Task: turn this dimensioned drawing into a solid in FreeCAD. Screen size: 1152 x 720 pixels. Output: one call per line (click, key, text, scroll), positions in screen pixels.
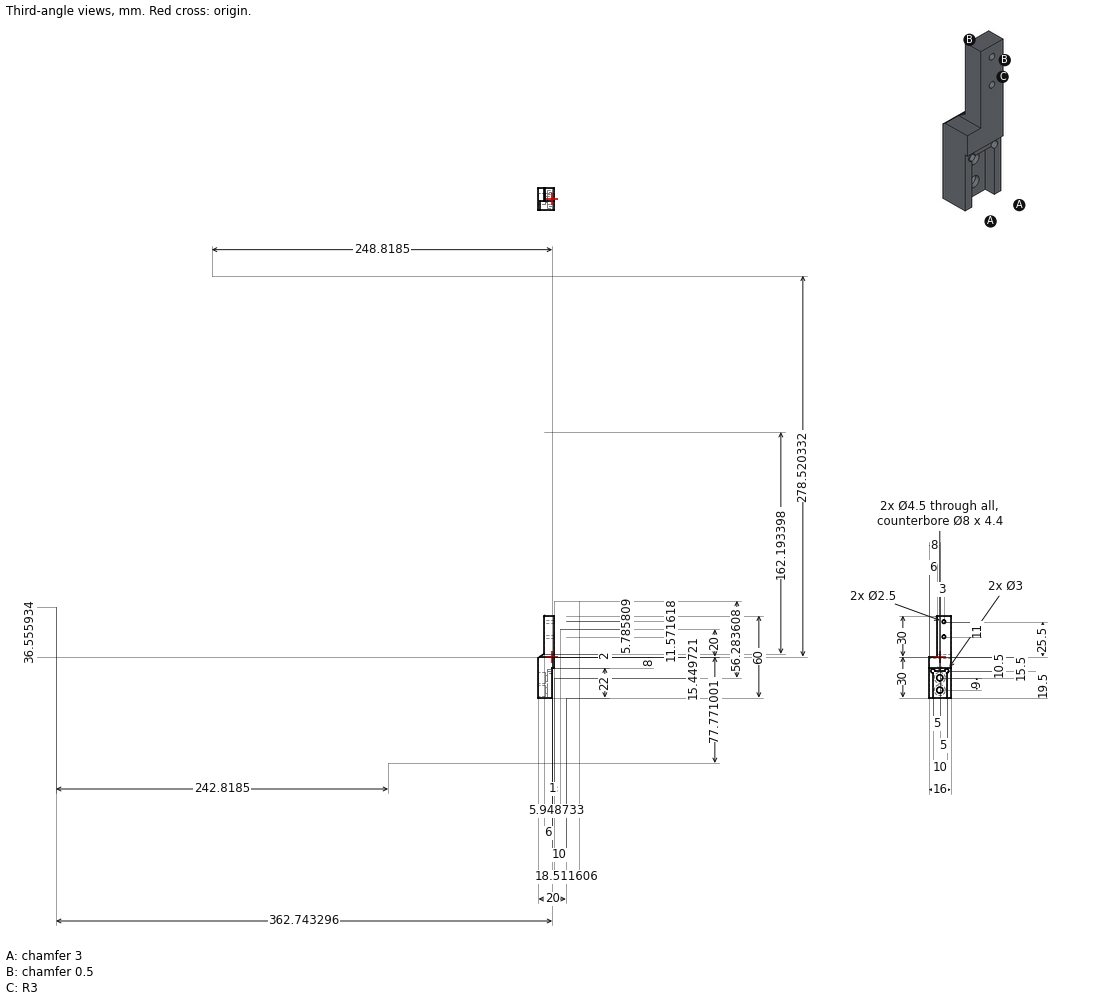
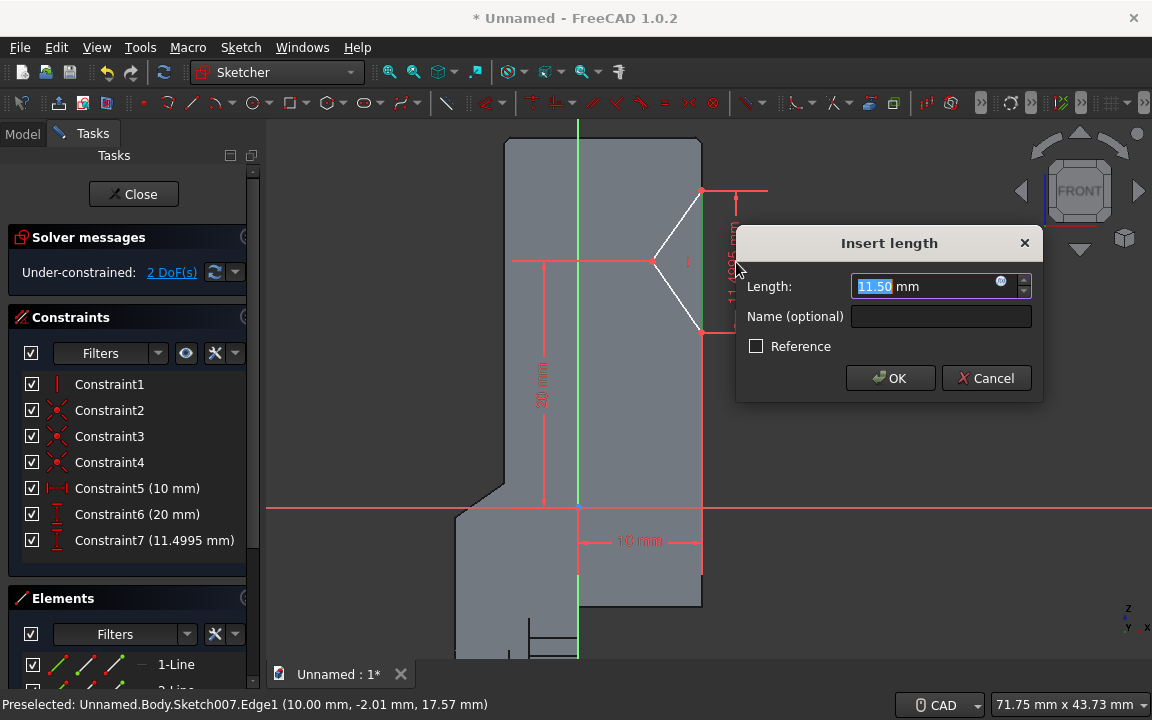
text(11.571618)
key(Return)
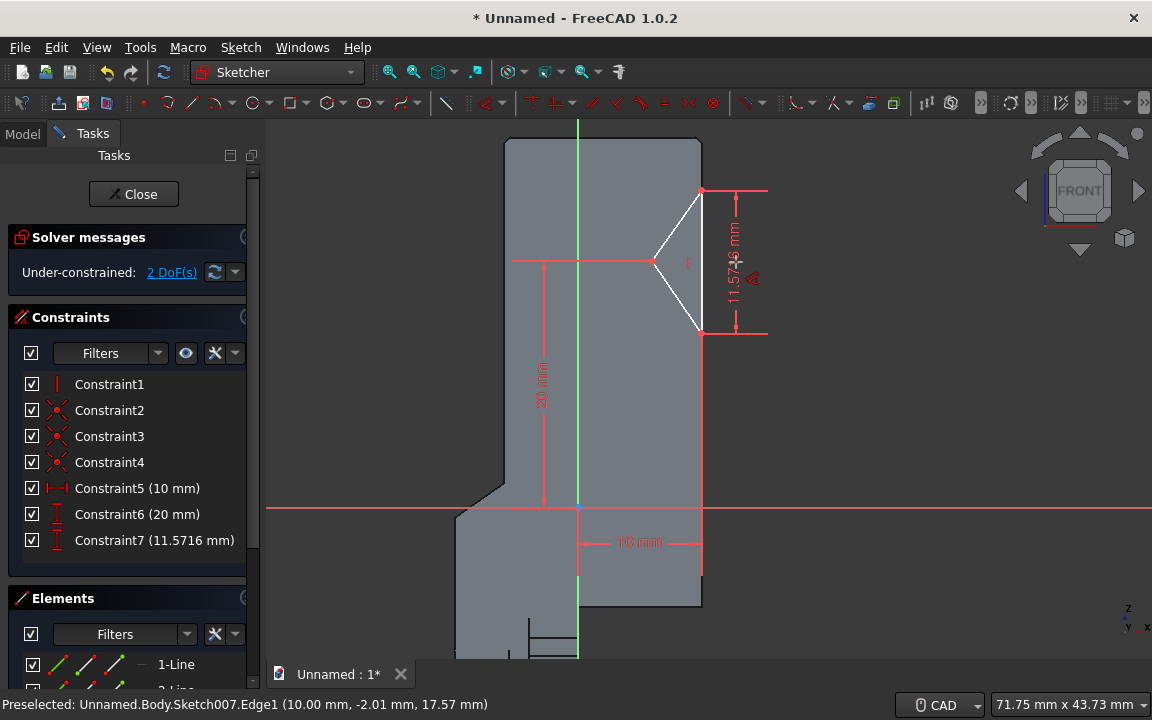
click(652, 261)
click(615, 227)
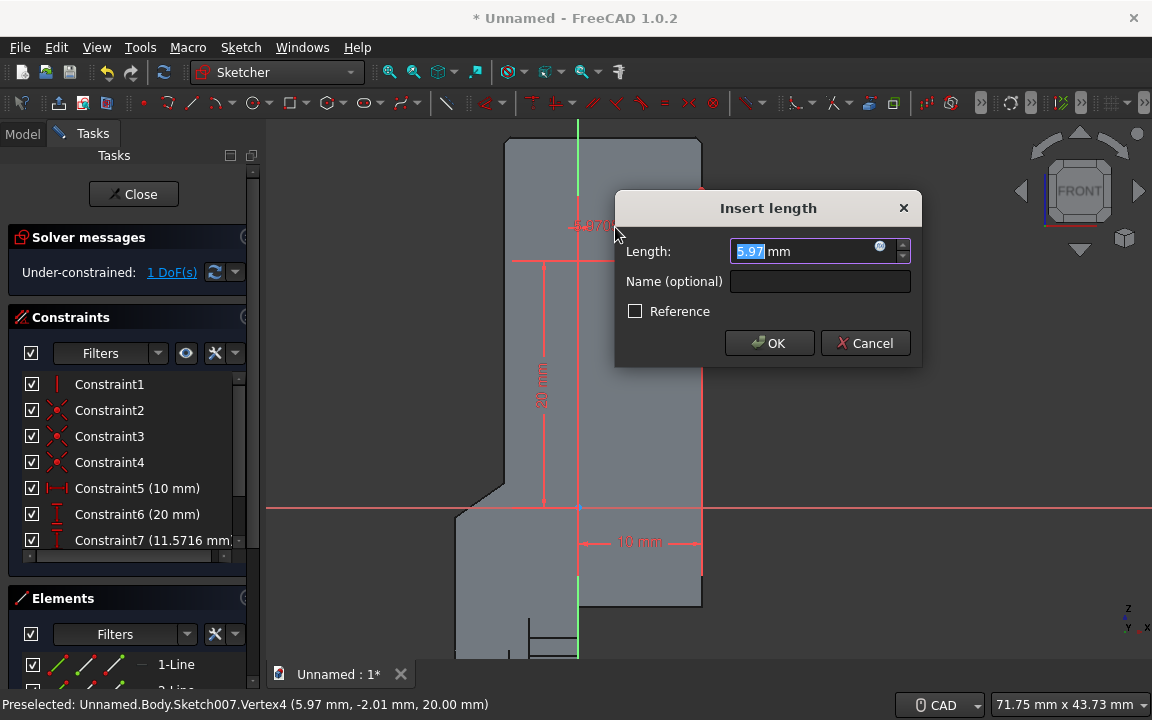
text(5.948733)
key(Return)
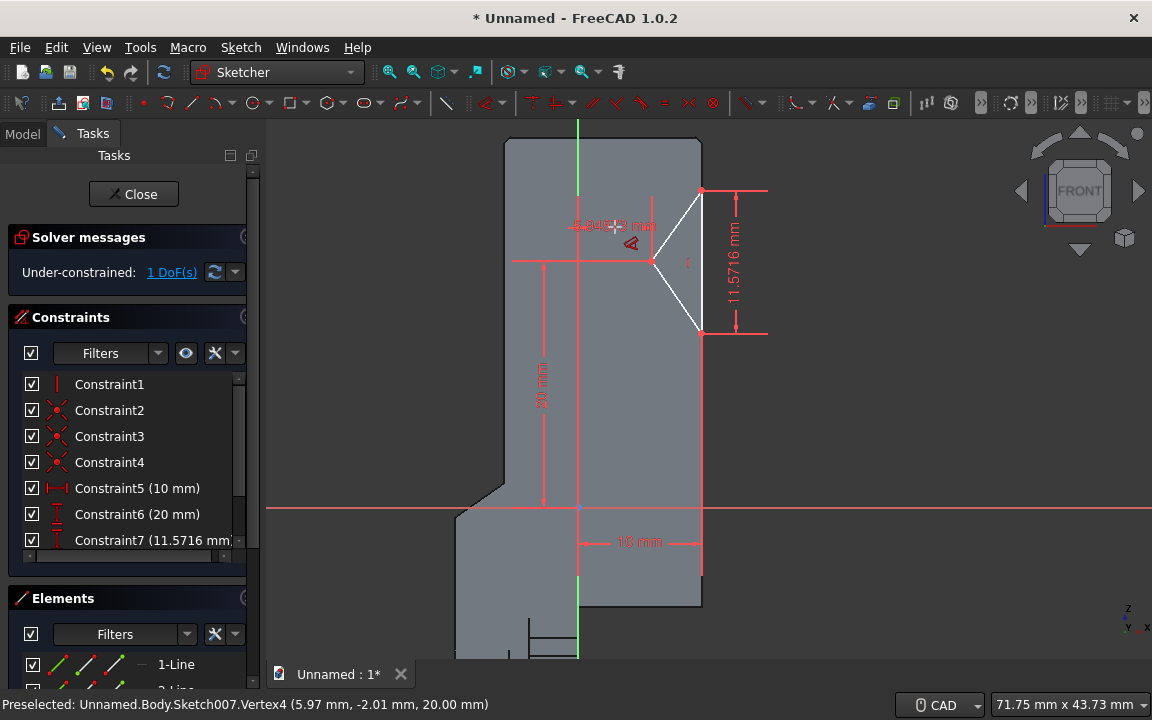
click(687, 212)
click(736, 226)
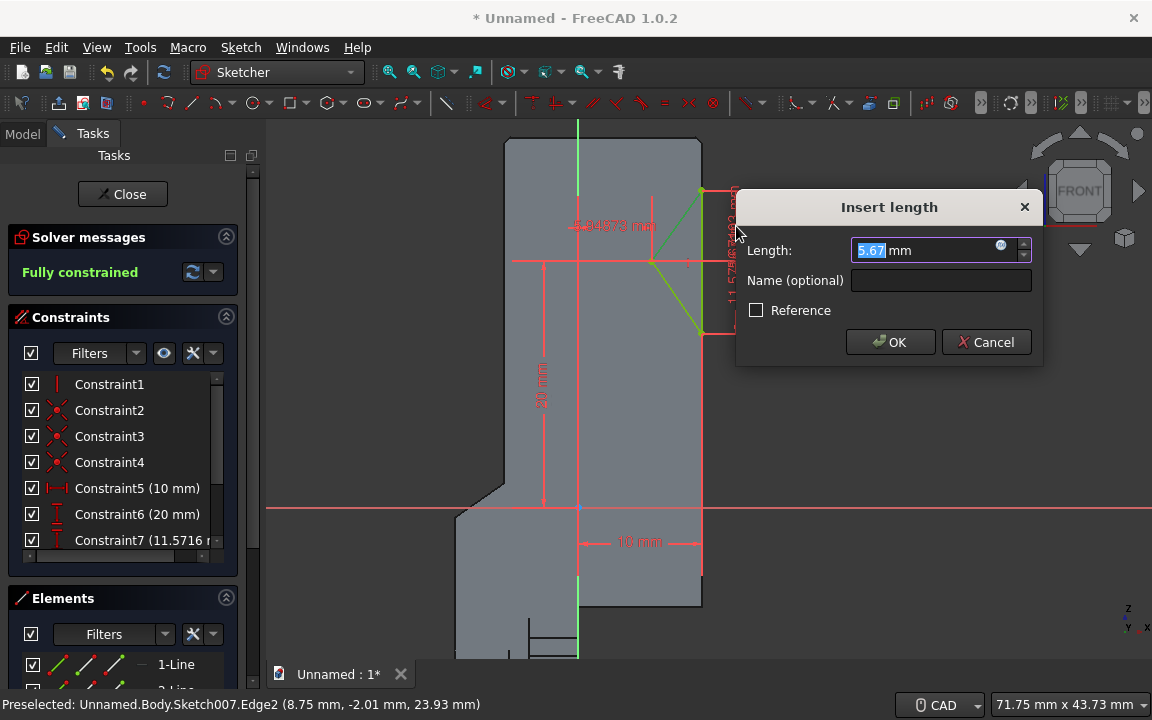
text(5.785809)
key(Return)
key(Escape)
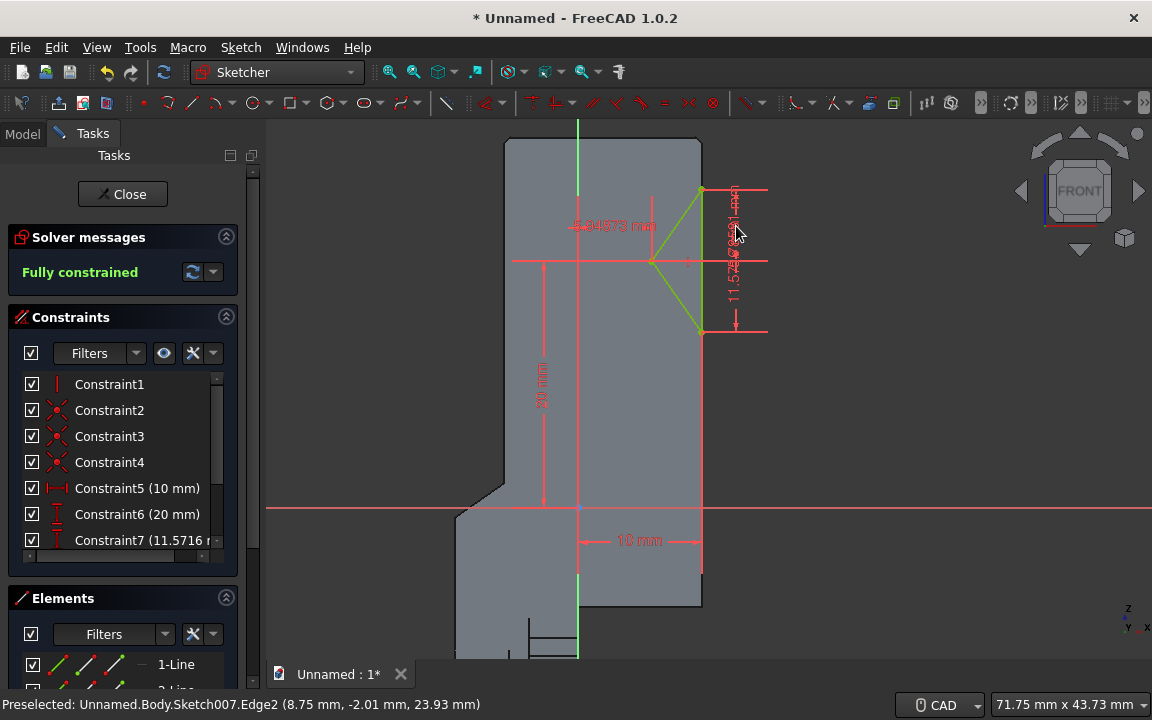
click(123, 194)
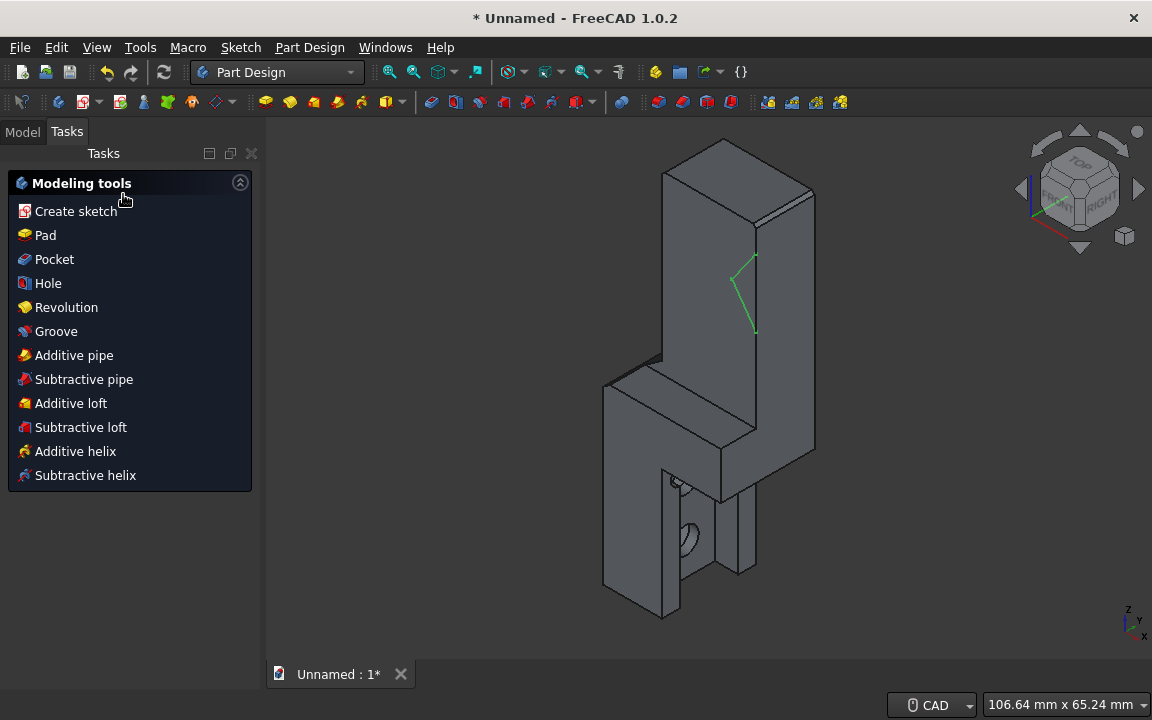
click(432, 102)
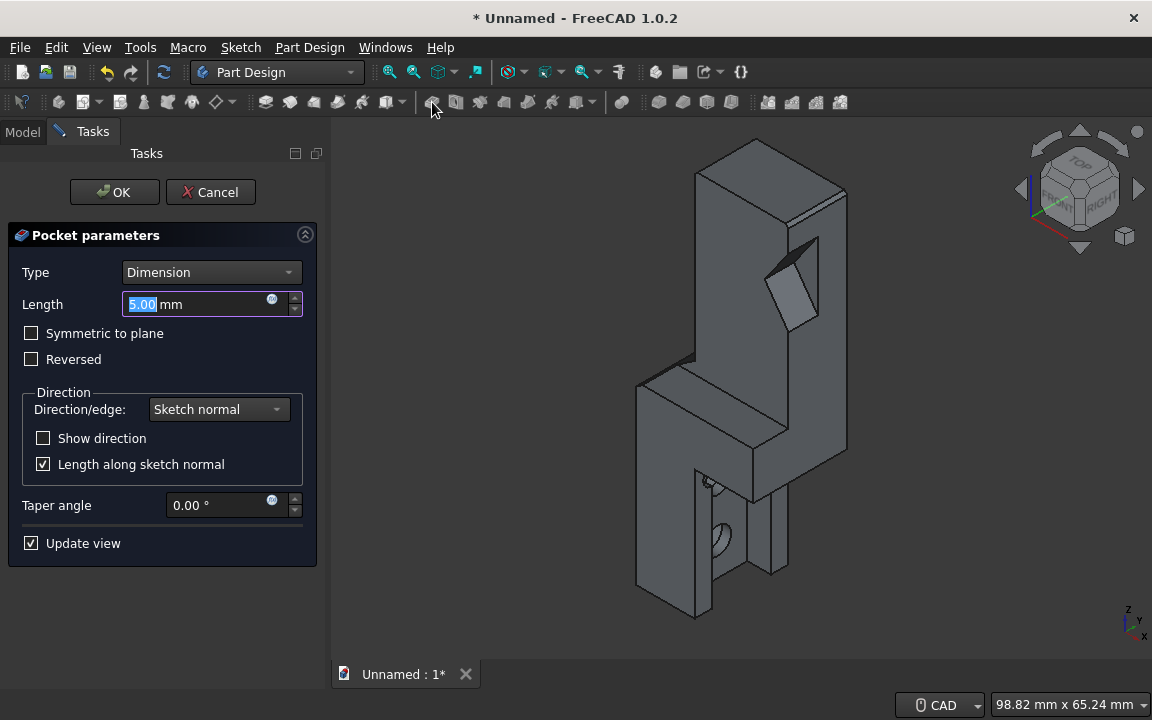
click(212, 272)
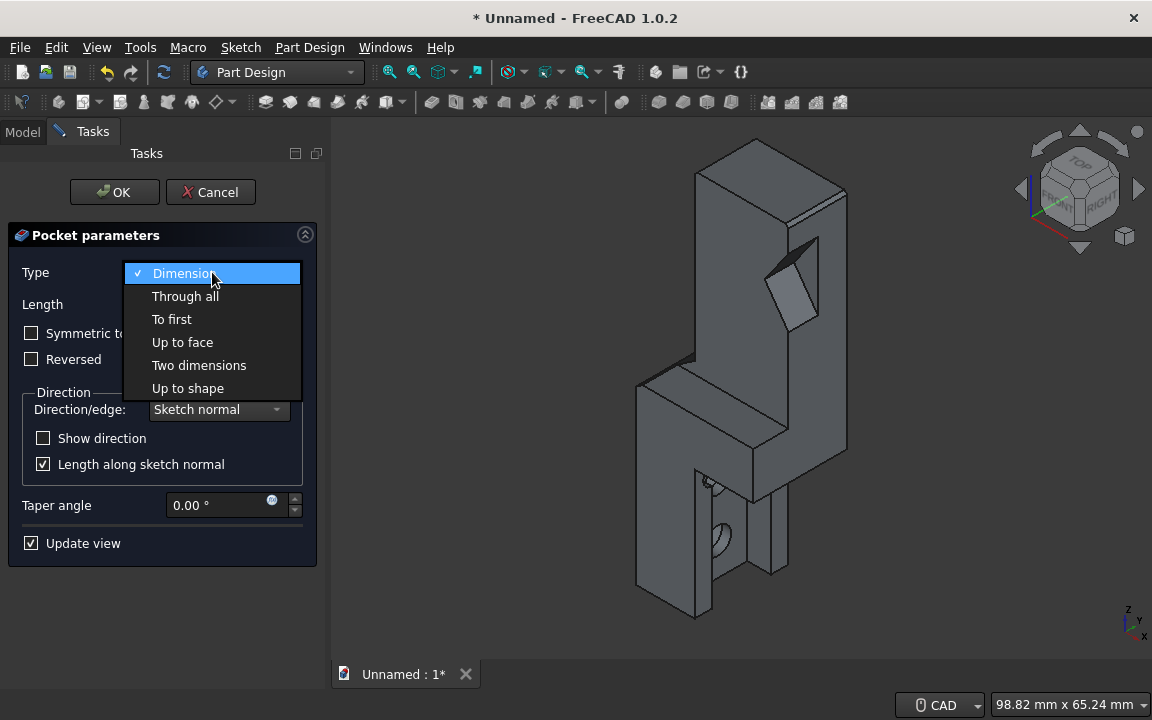
click(212, 296)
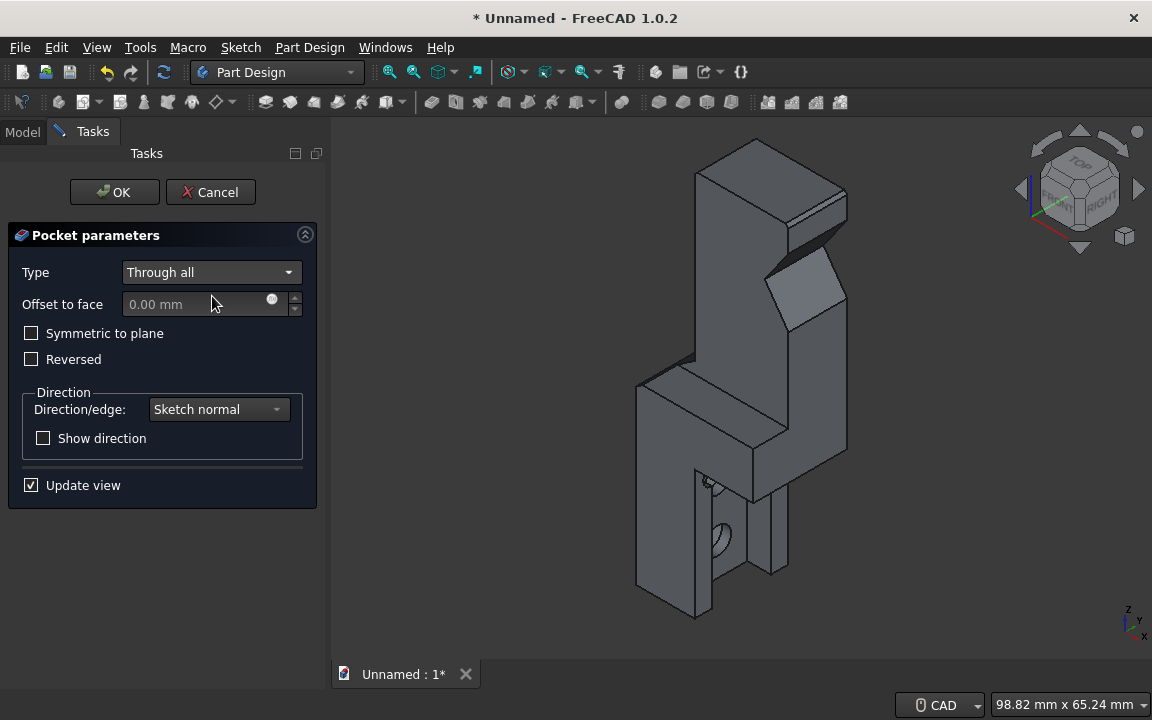
click(115, 192)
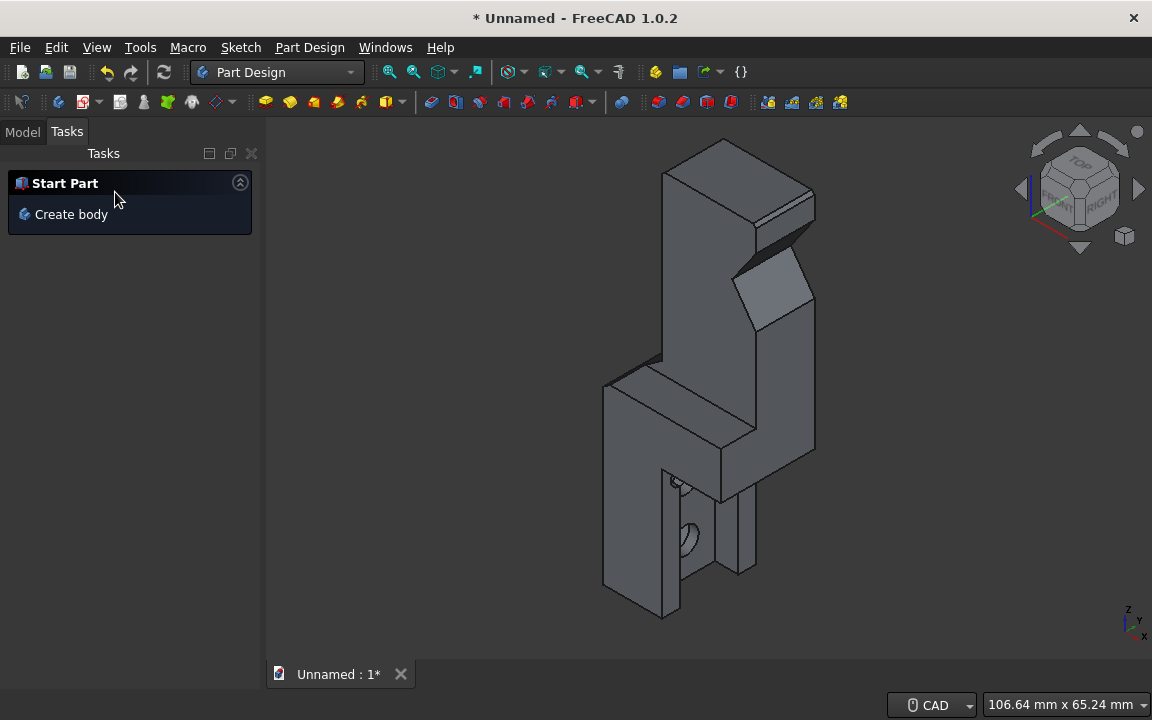
key(2)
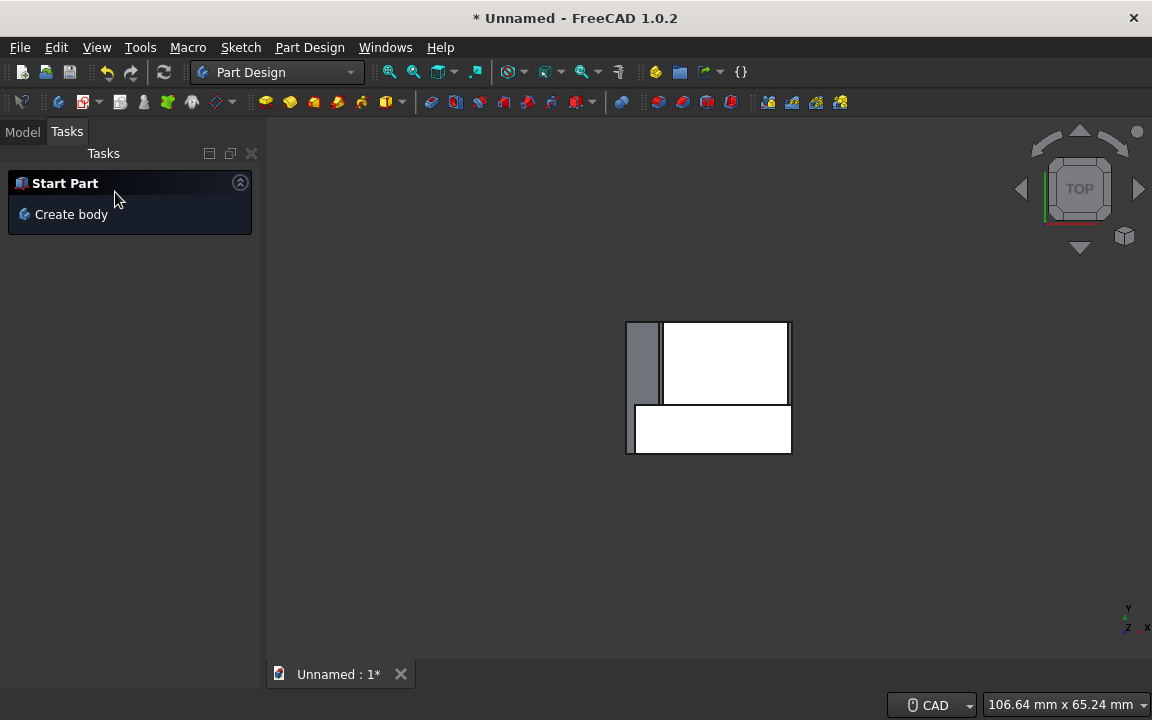
click(390, 72)